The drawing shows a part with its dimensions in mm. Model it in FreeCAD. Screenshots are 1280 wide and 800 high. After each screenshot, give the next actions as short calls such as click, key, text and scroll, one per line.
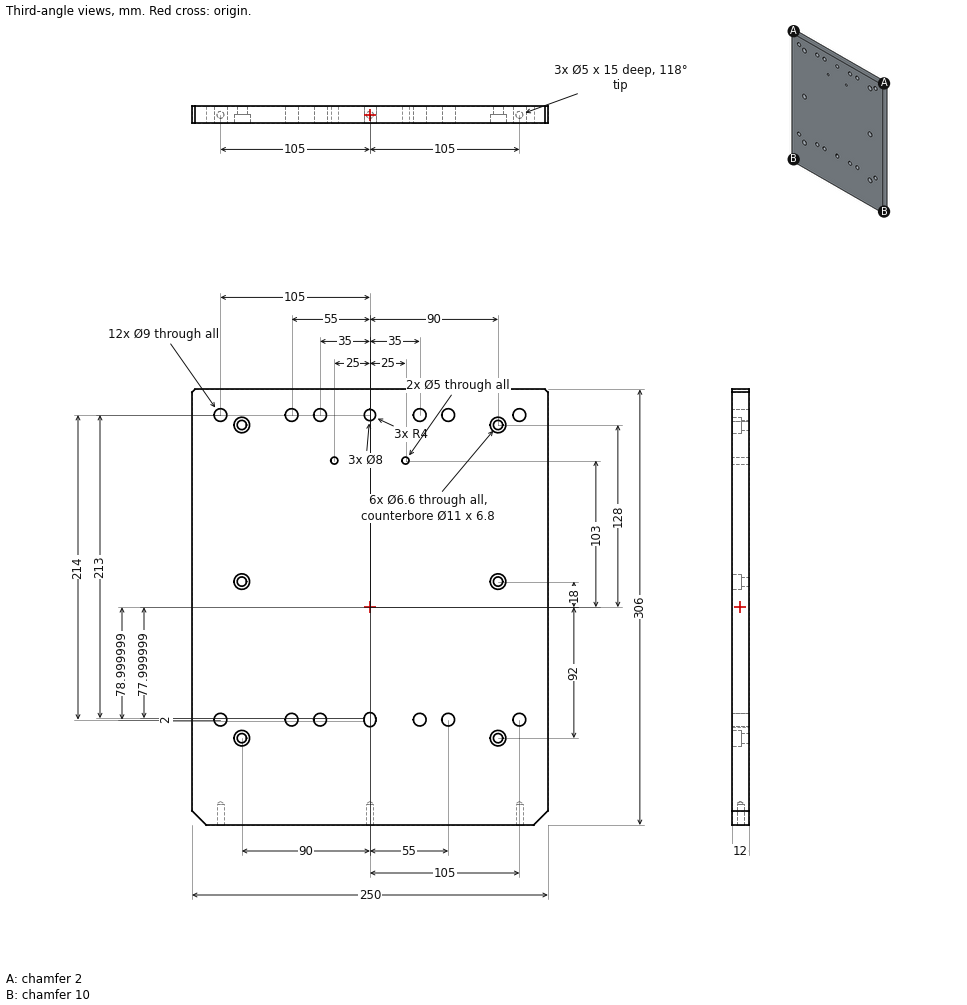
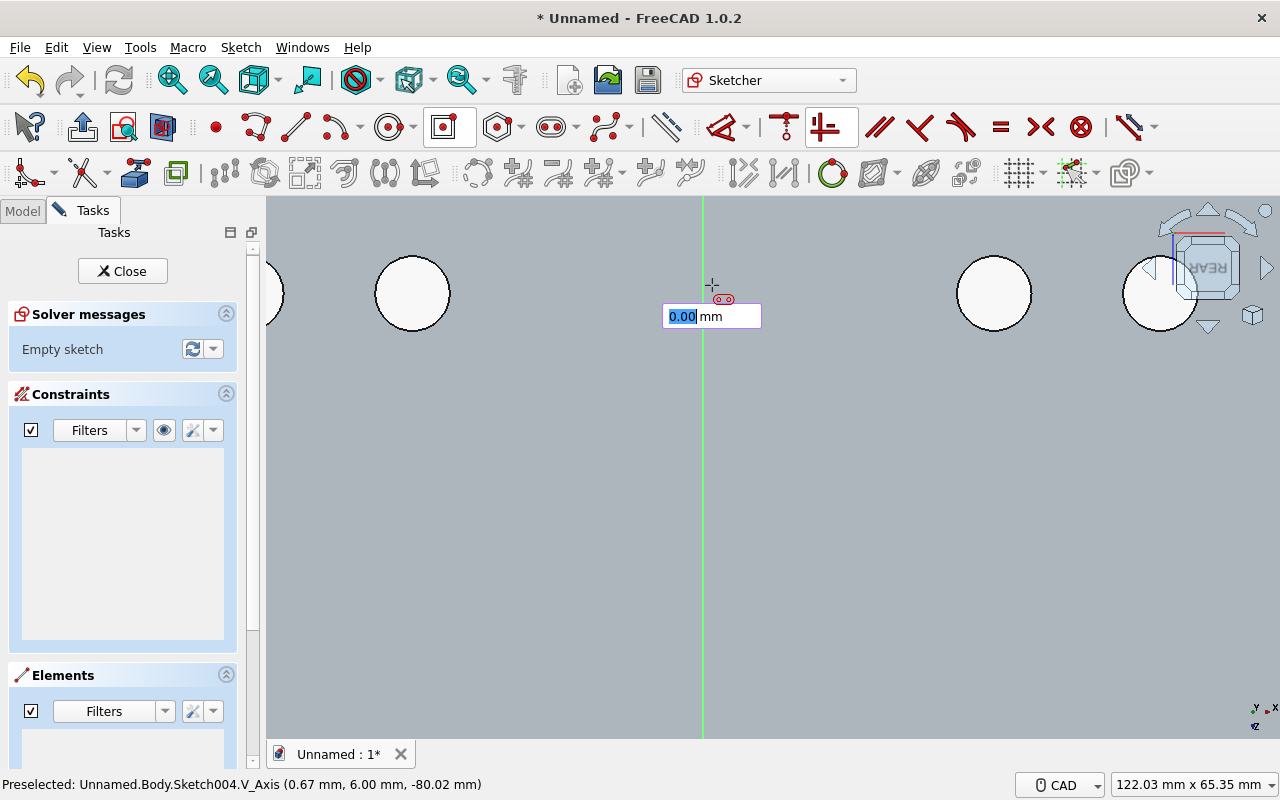
click(670, 294)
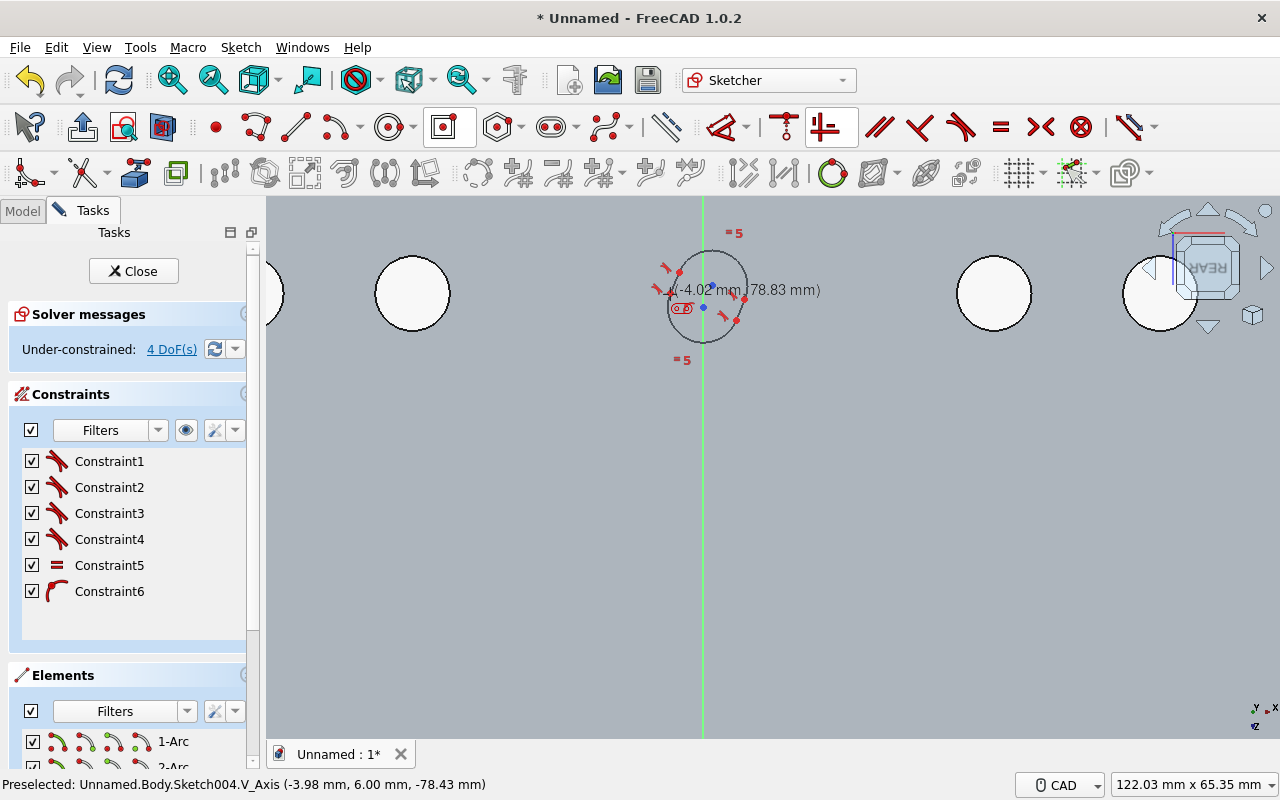
click(390, 128)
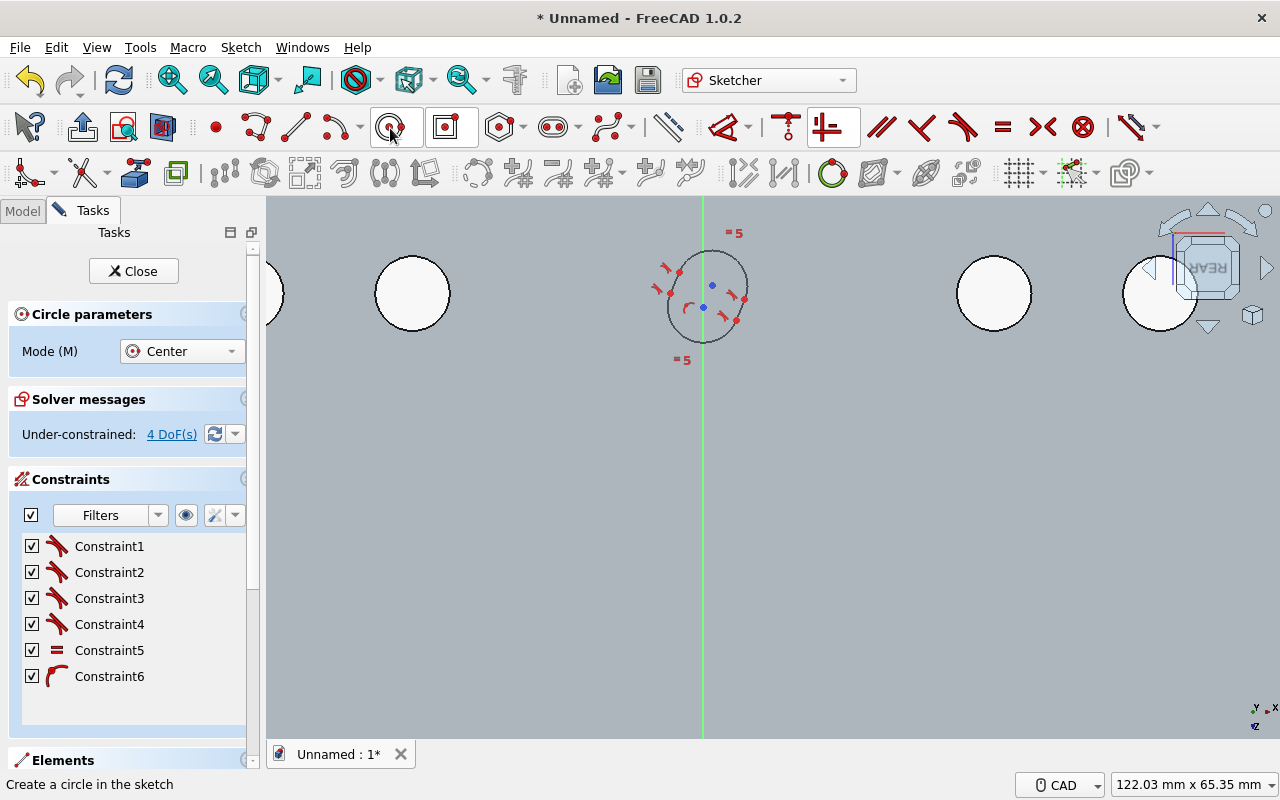
scroll(705, 288, down, 8)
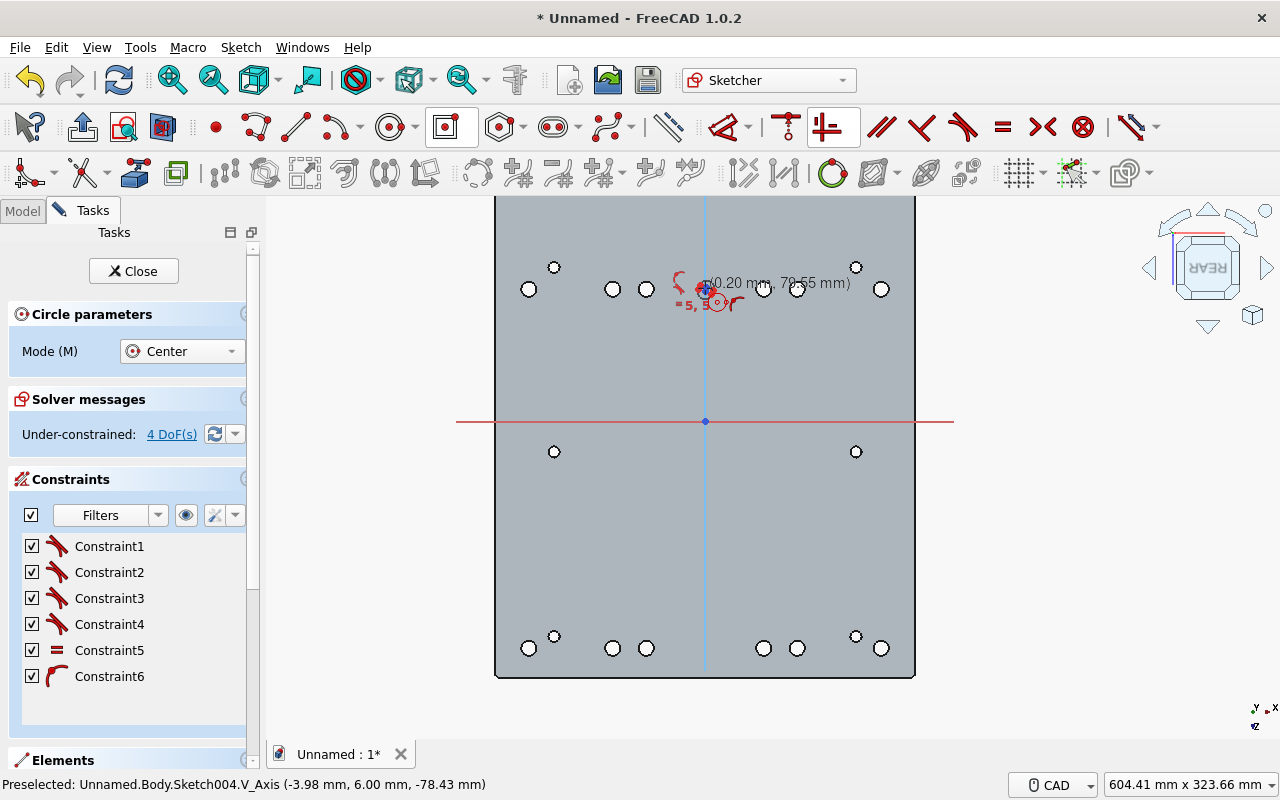
scroll(705, 648, up, 7)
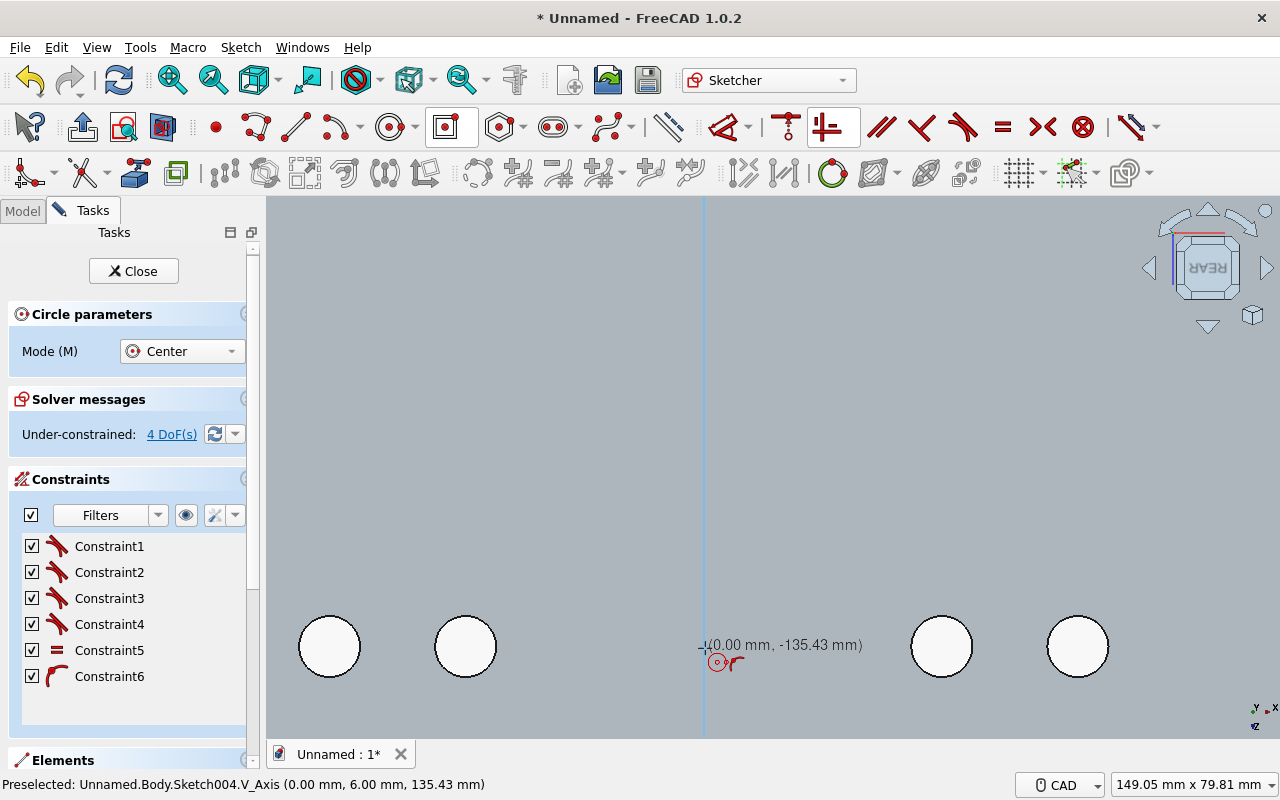
scroll(705, 648, down, 7)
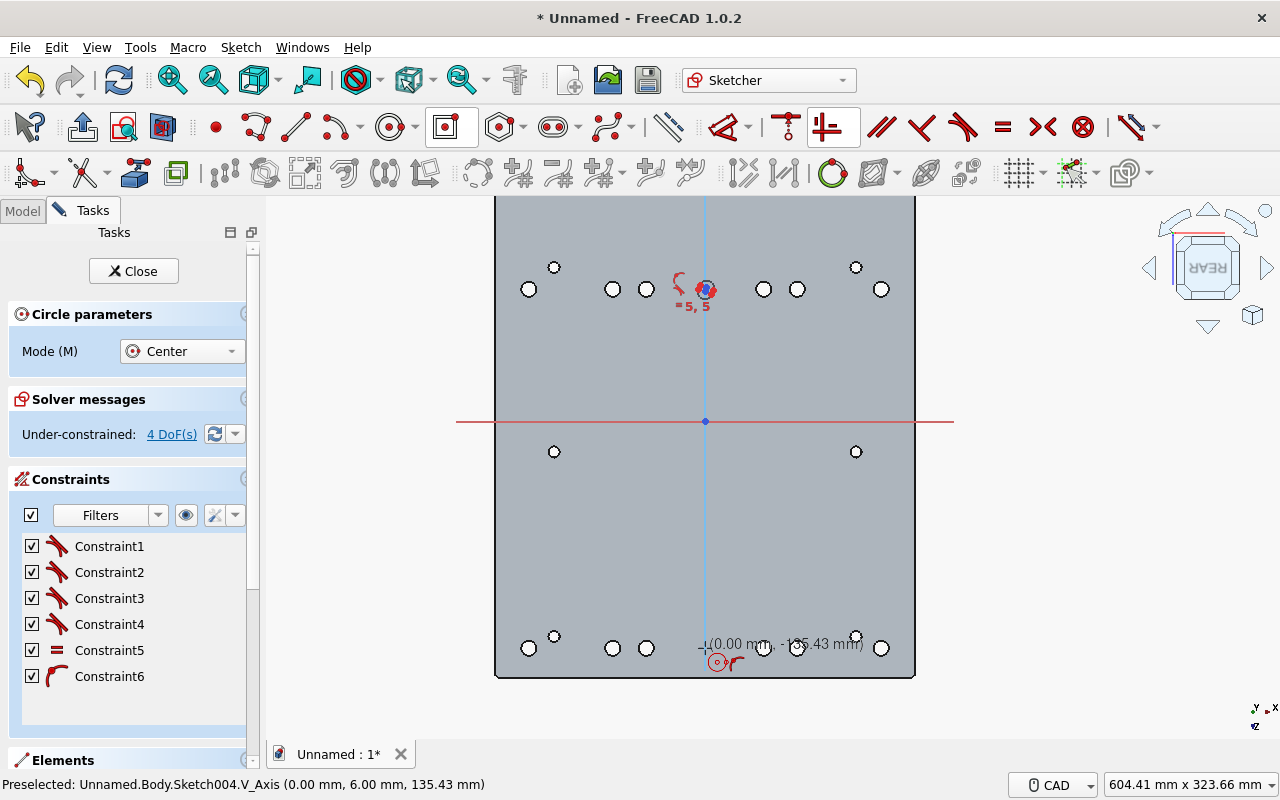
click(705, 648)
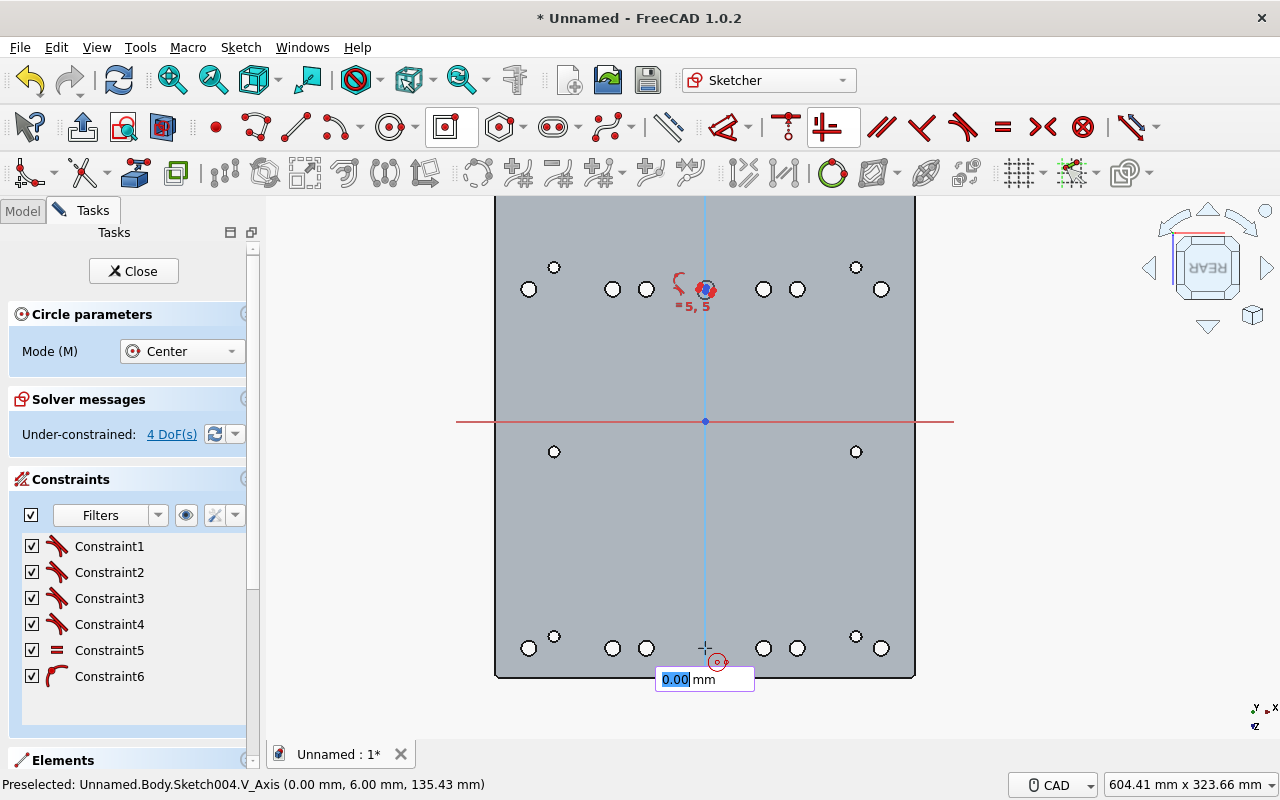
scroll(711, 646, up, 5)
move(711, 645)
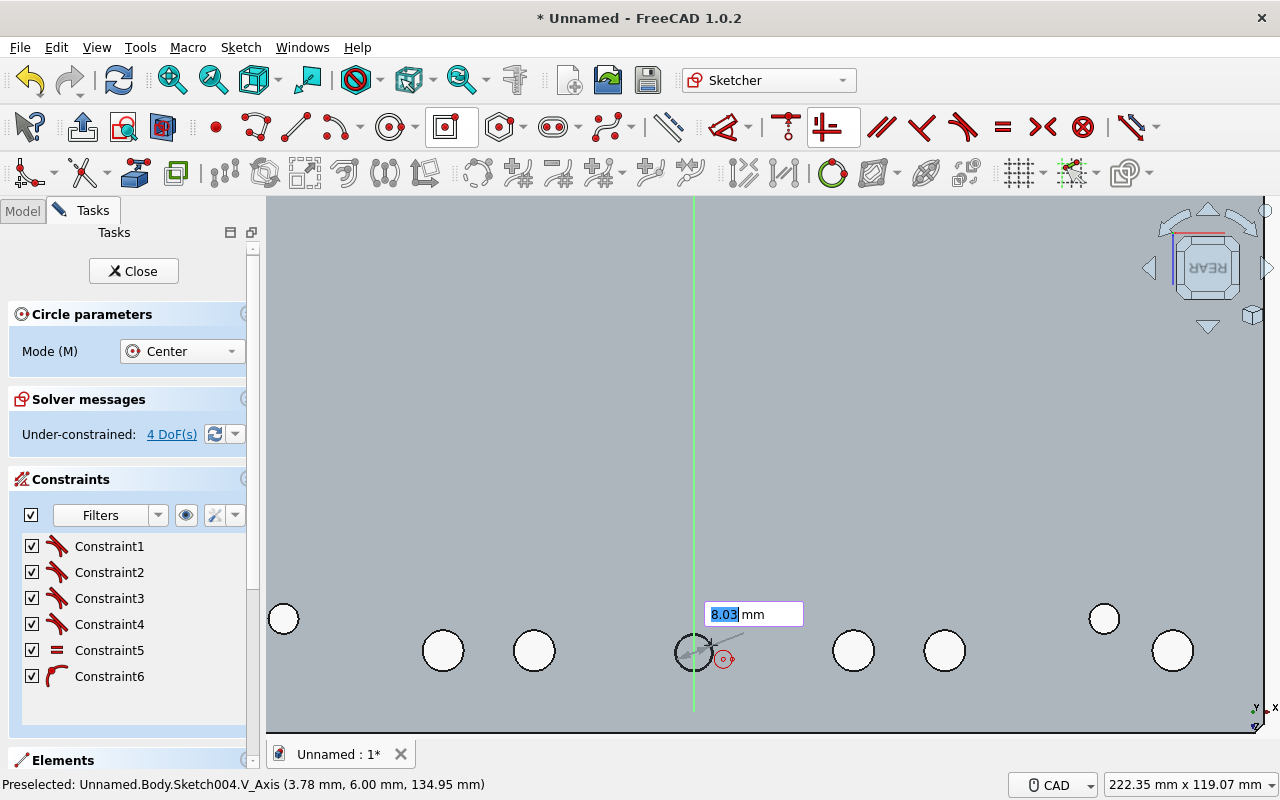
text(8)
key(Return)
key(Escape)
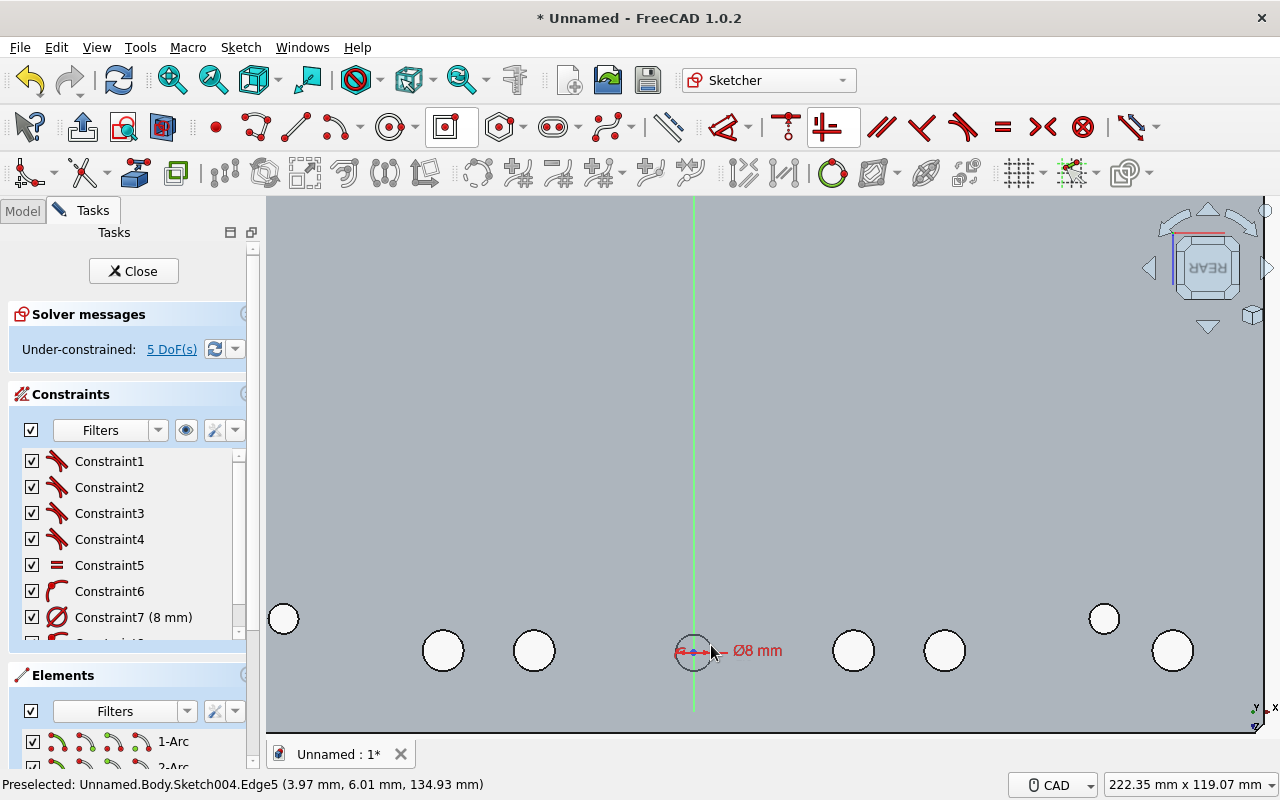
scroll(711, 646, down, 5)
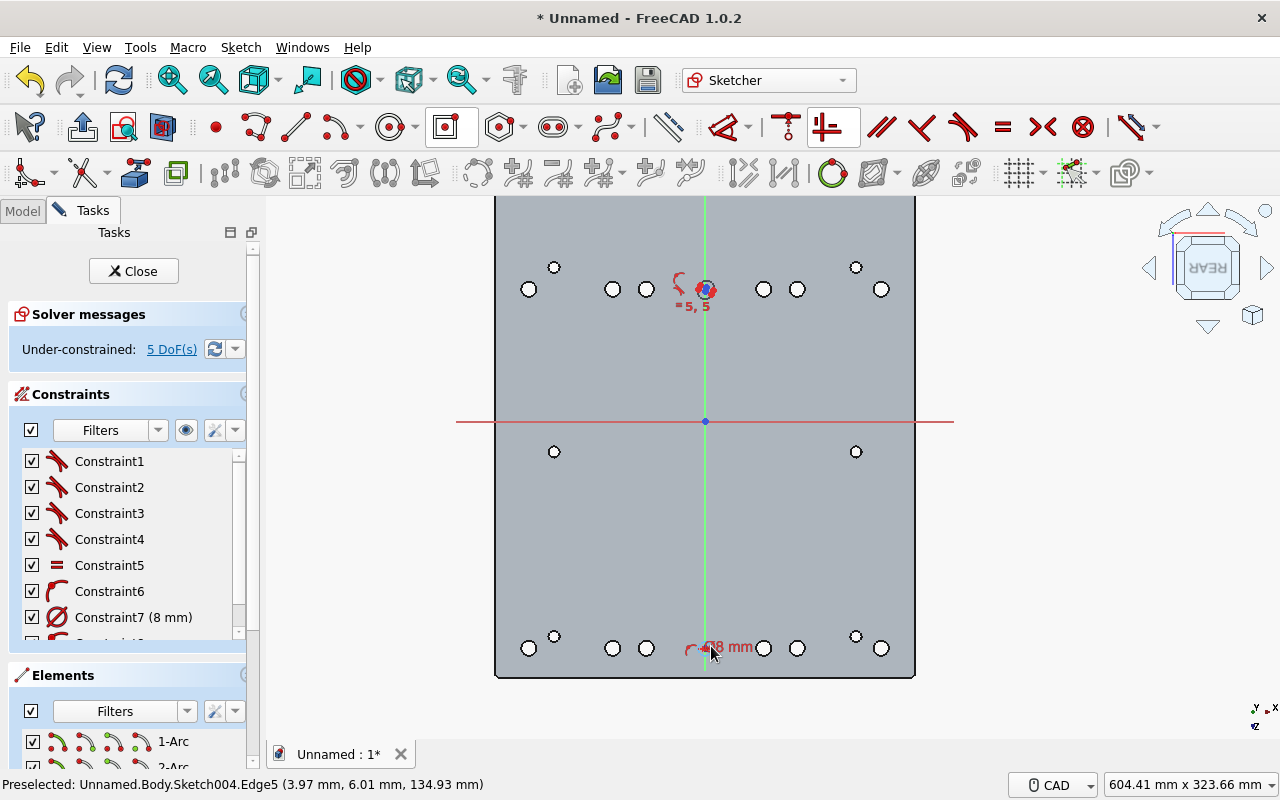
scroll(707, 288, up, 5)